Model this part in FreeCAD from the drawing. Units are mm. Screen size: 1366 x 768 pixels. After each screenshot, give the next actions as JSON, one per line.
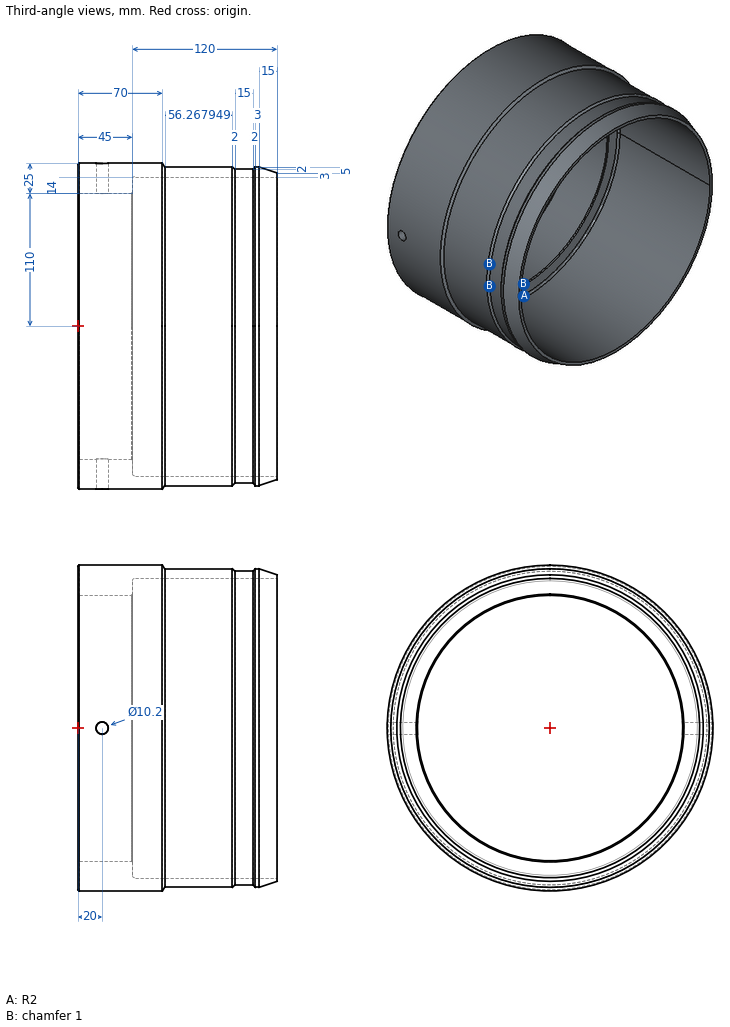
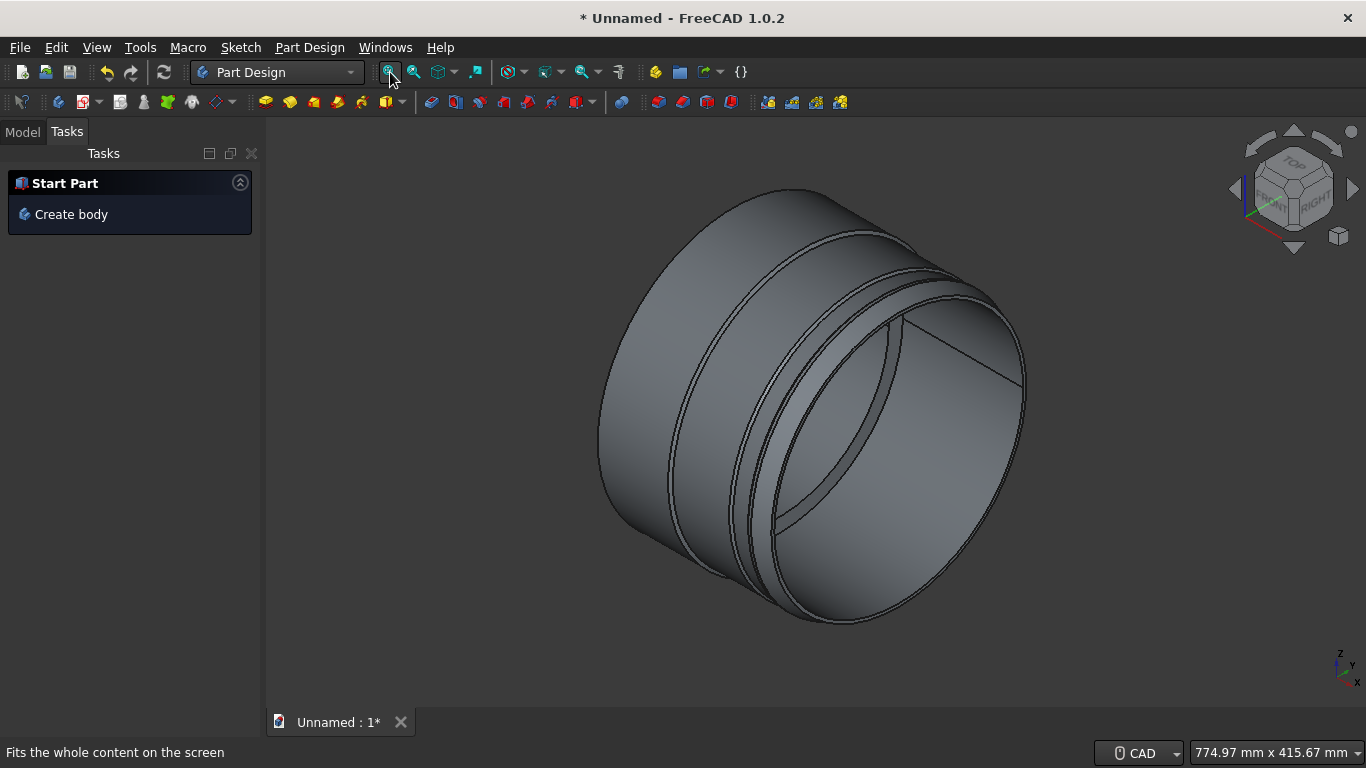
{"action": "key", "text": "2"}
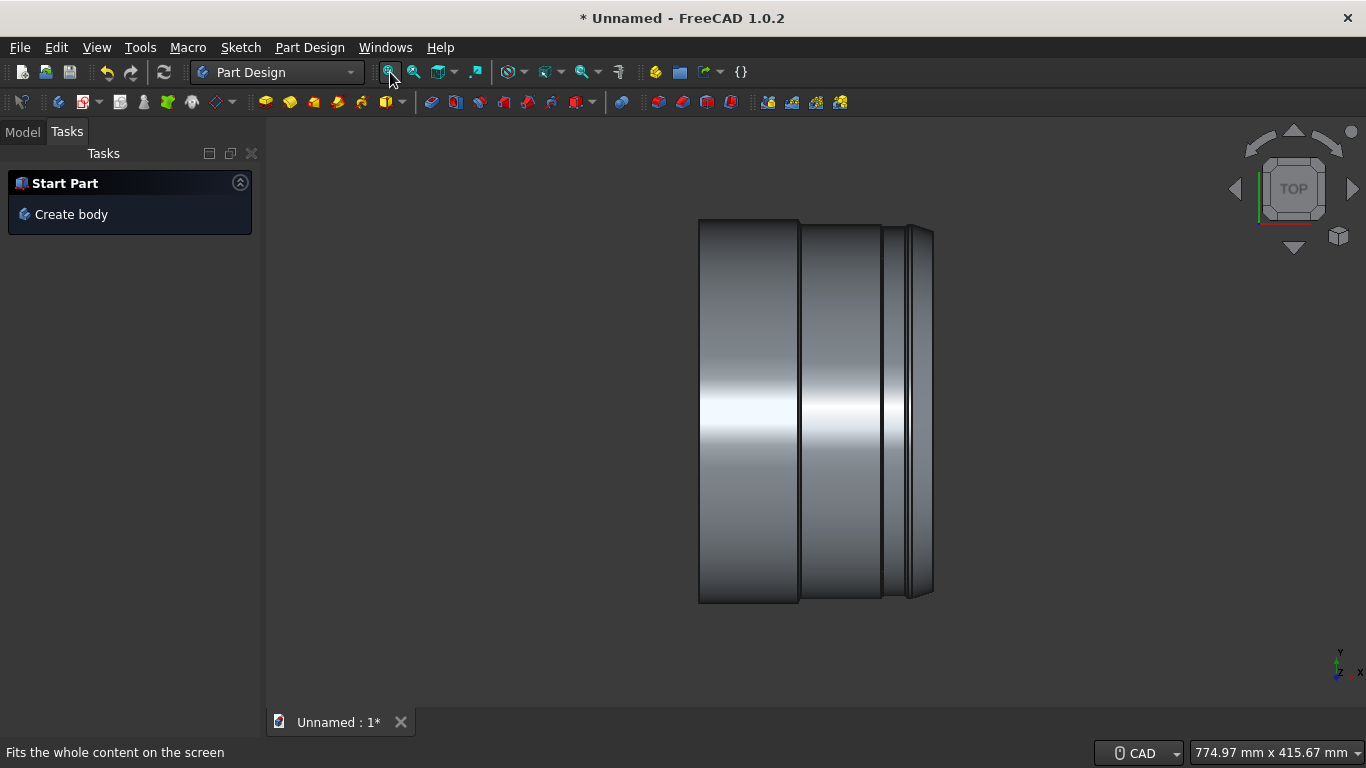
{"action": "key", "text": "1"}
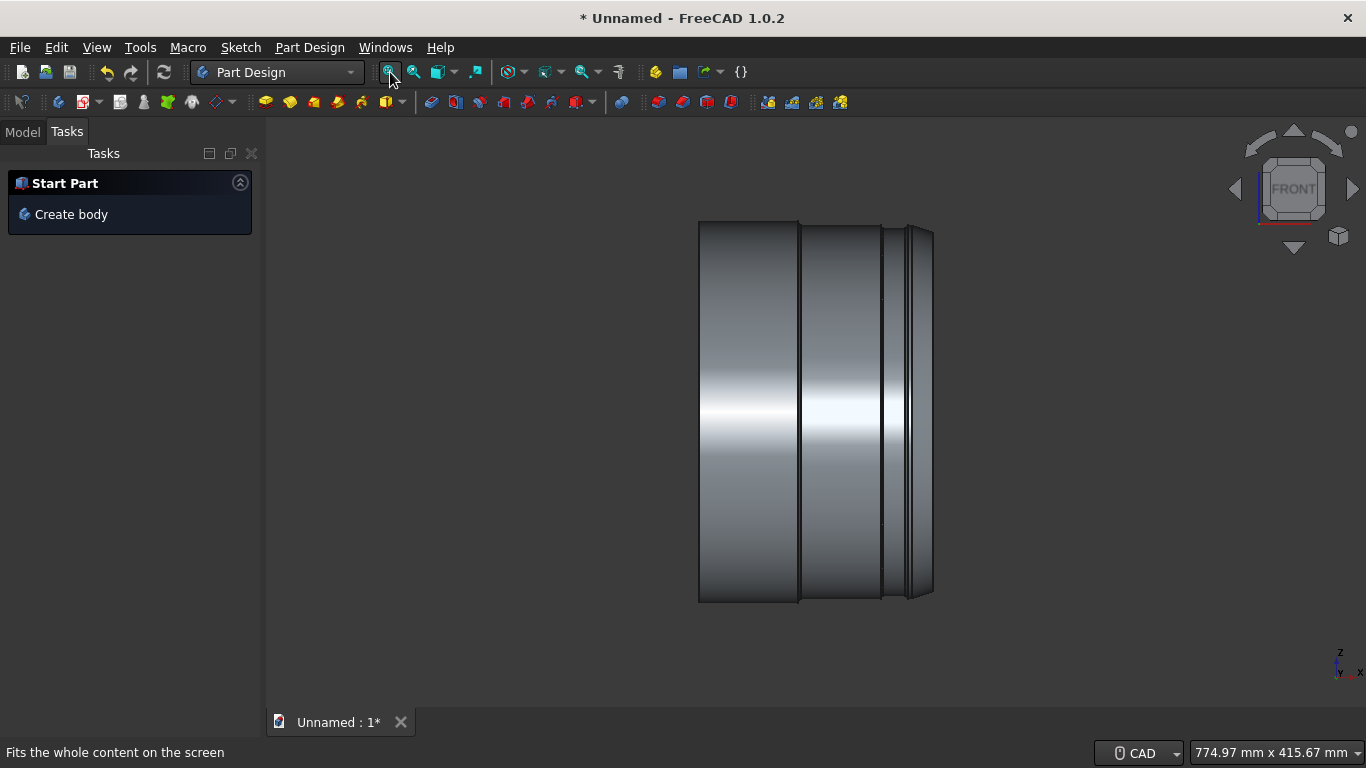
{"action": "key", "text": "3"}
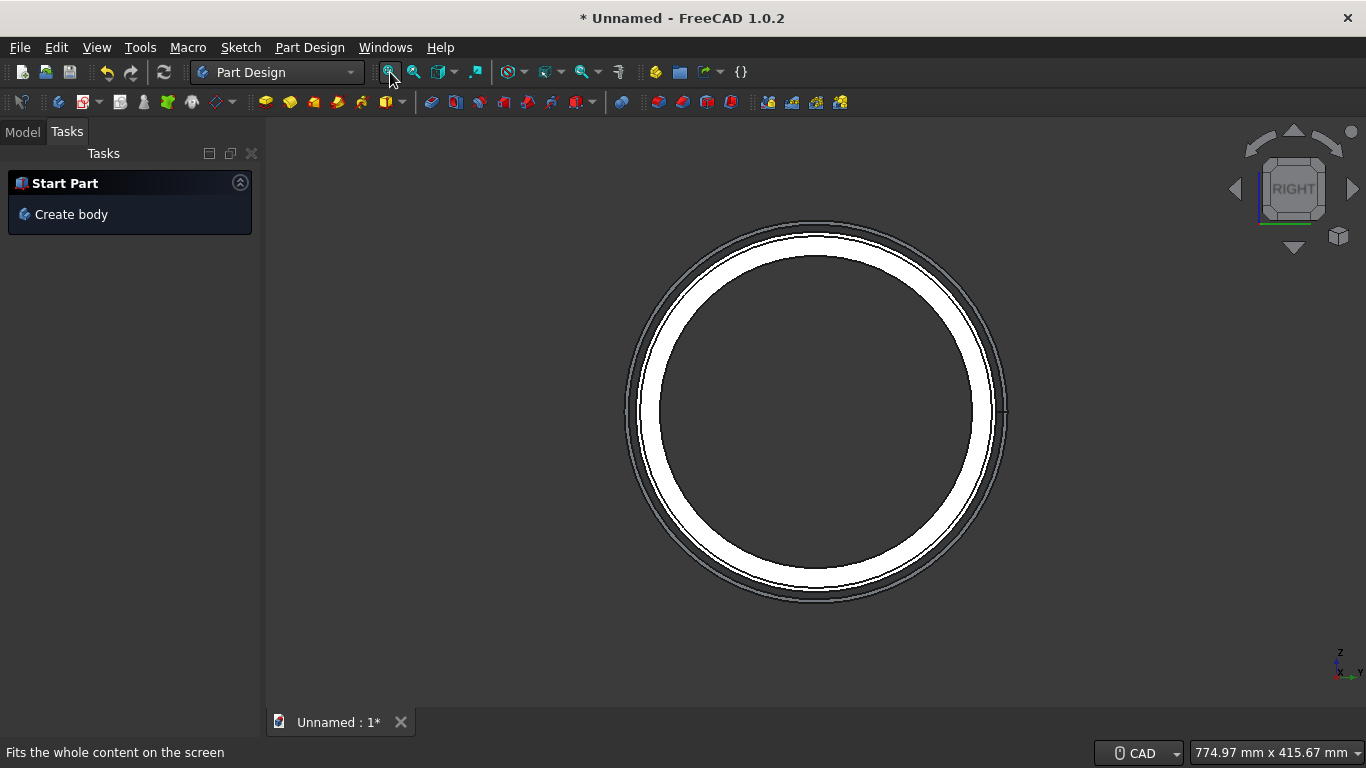
{"action": "key", "text": "5"}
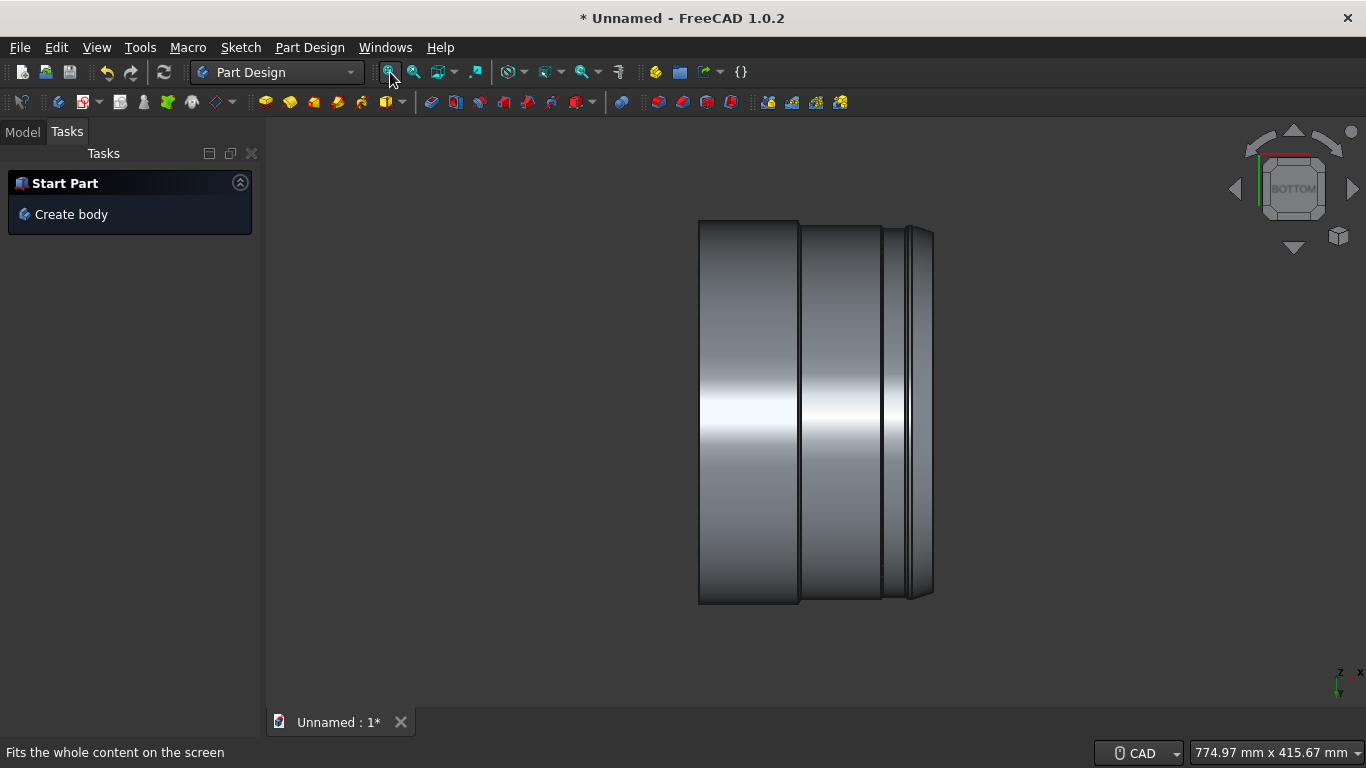
{"action": "key", "text": "4"}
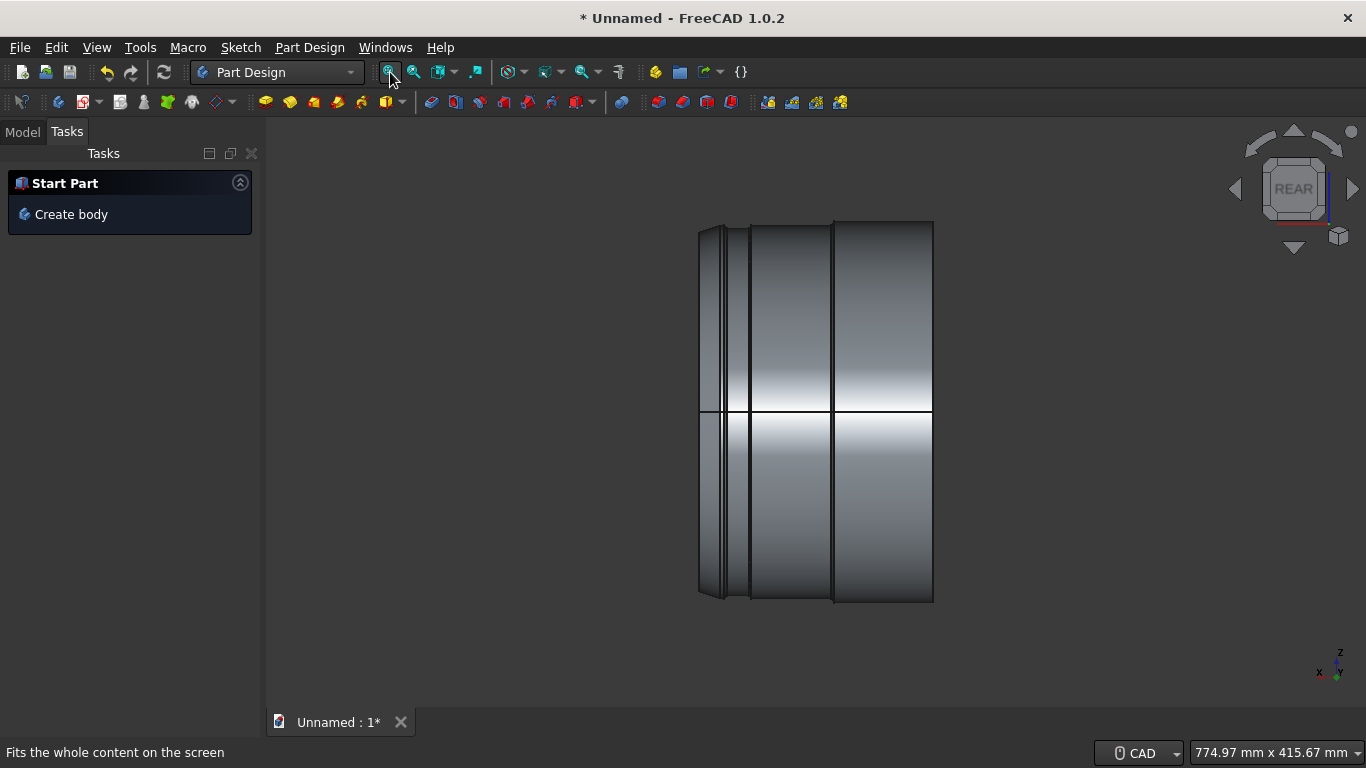
{"action": "key", "text": "6"}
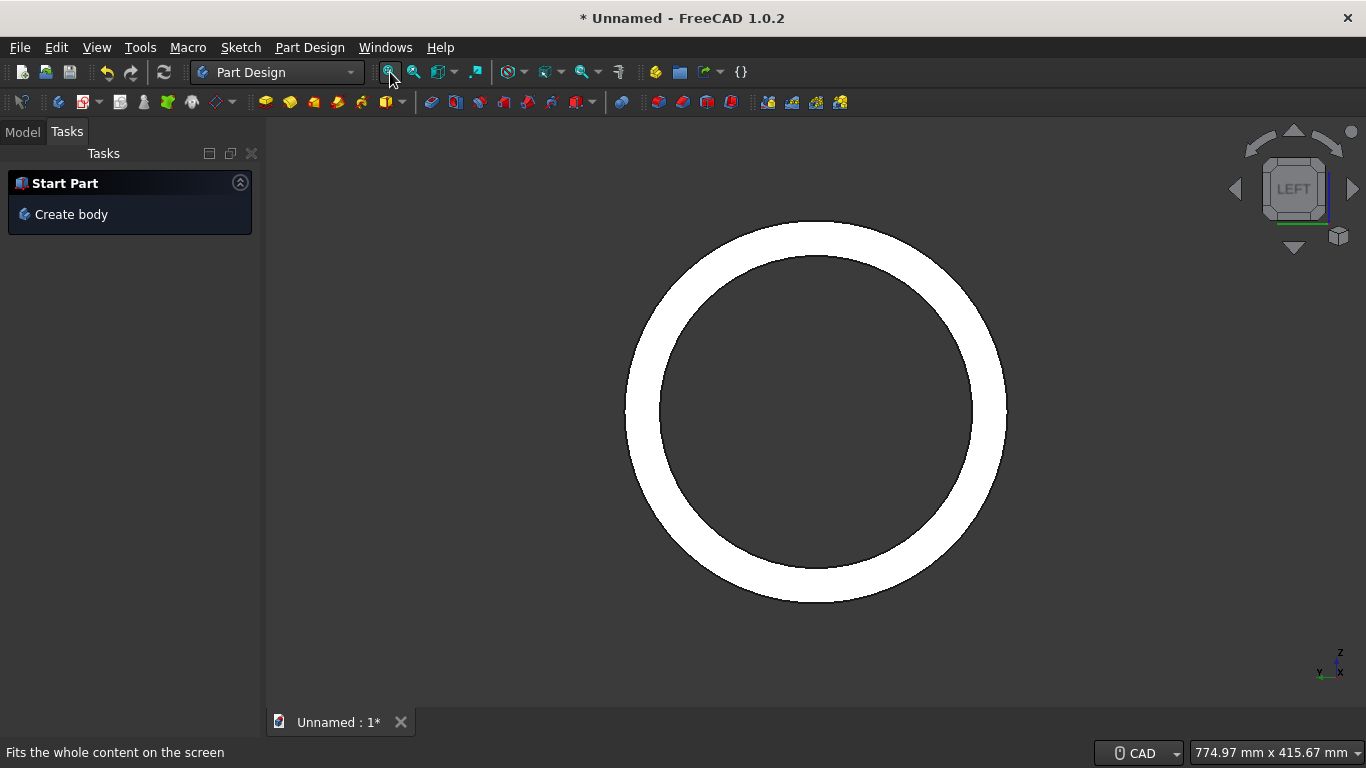
{"action": "key", "text": "v 3"}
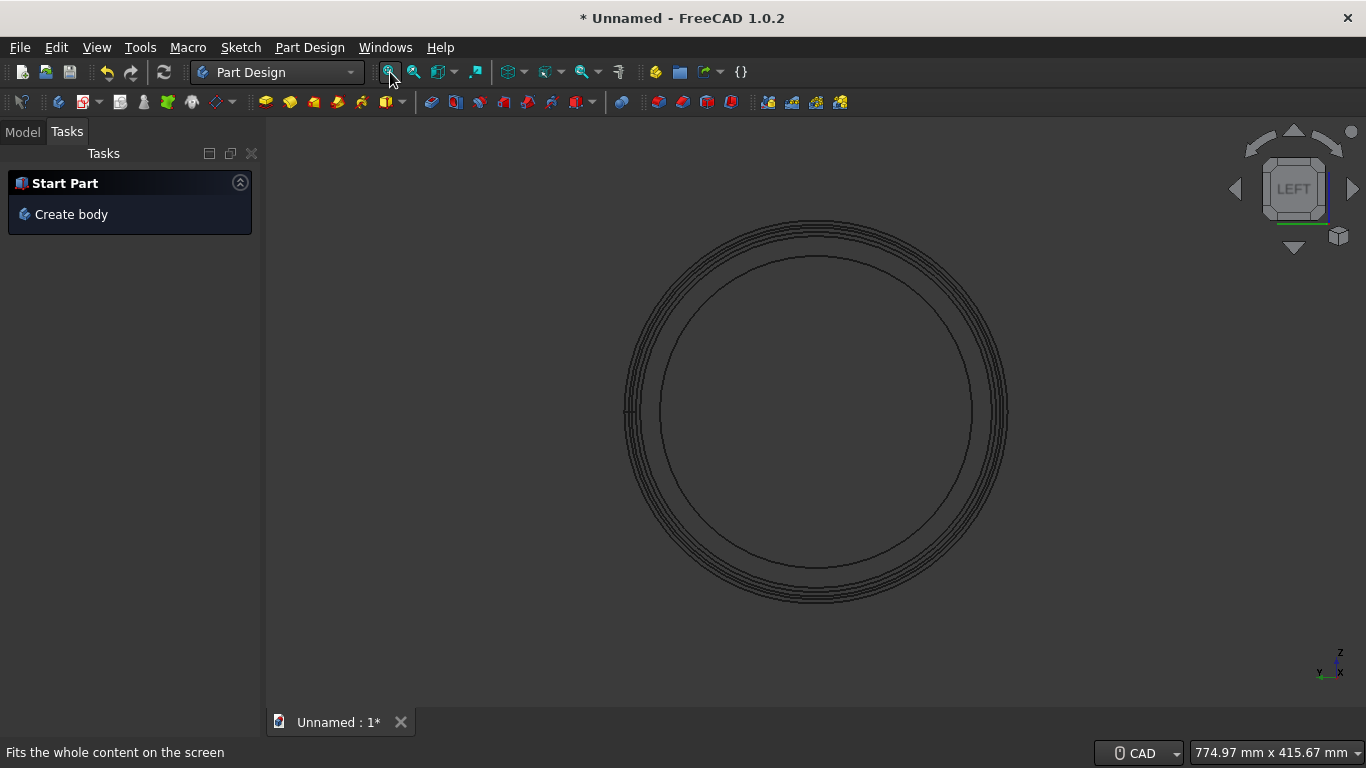
{"action": "key", "text": "0"}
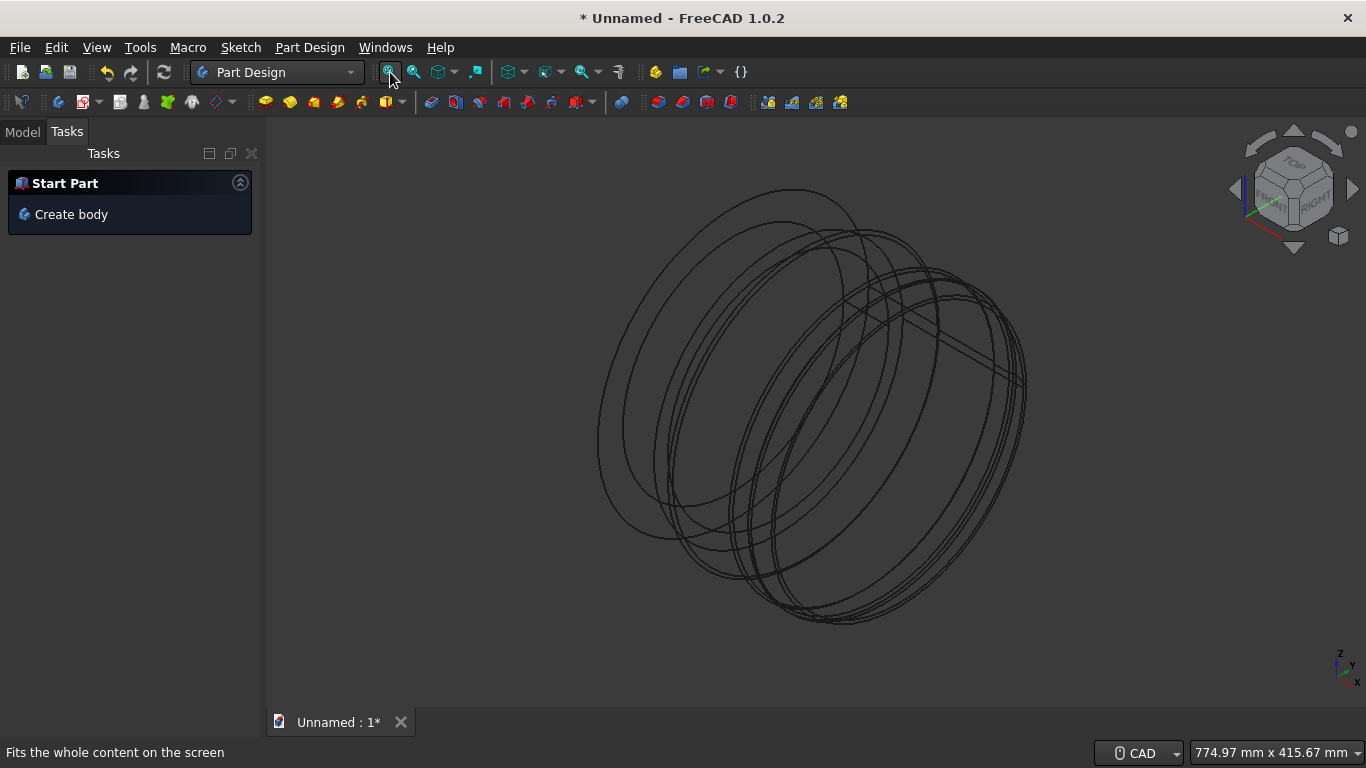
{"action": "left_click", "coordinate": [654, 461]}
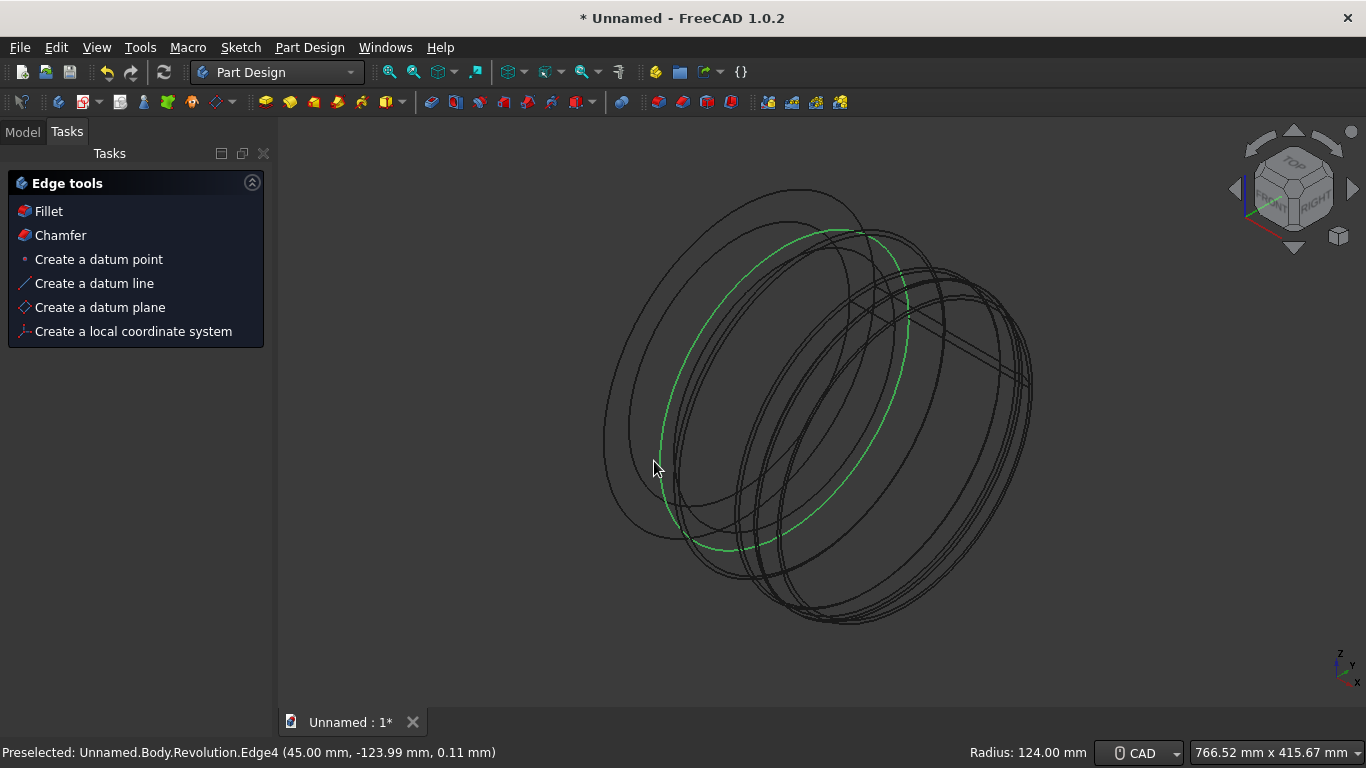
{"action": "key", "text": "v 1"}